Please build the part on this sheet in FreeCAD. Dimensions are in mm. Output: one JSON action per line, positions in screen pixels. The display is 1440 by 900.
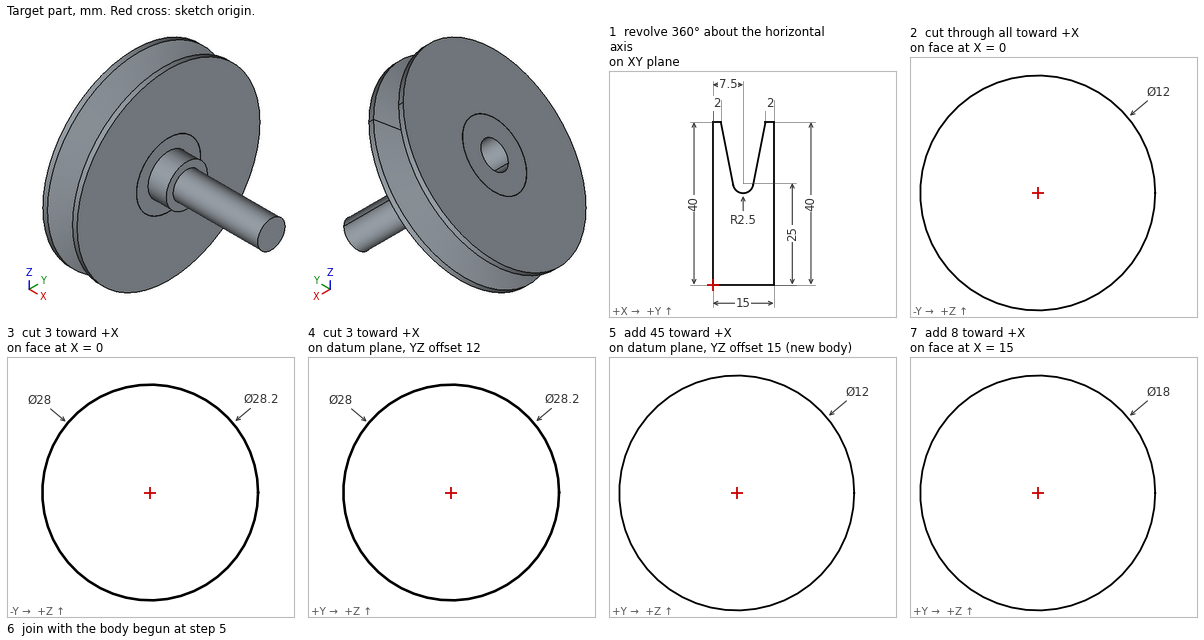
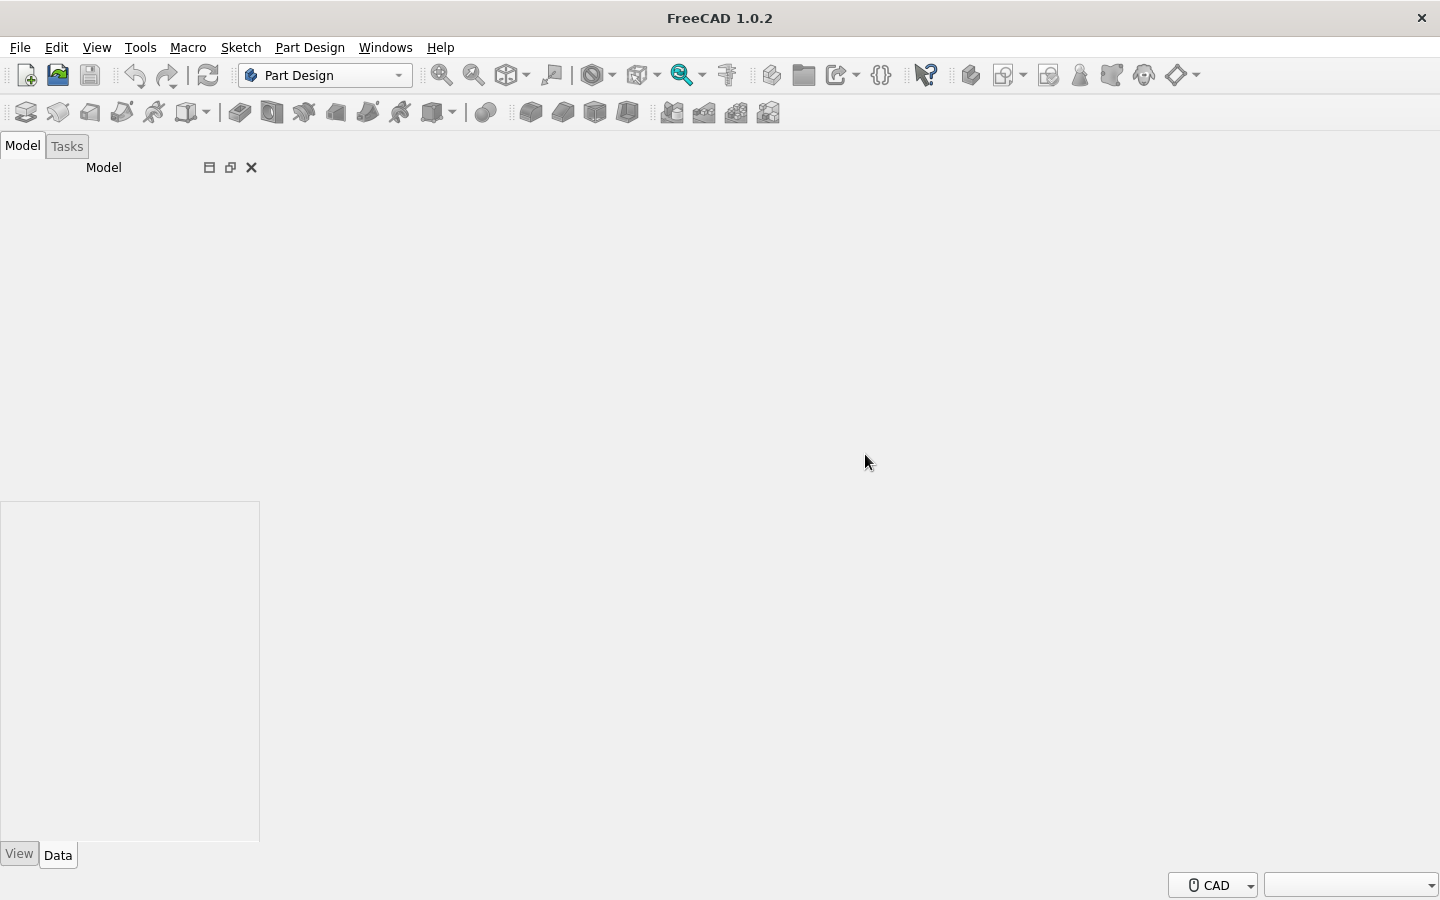
{"action": "left_click", "coordinate": [26, 76]}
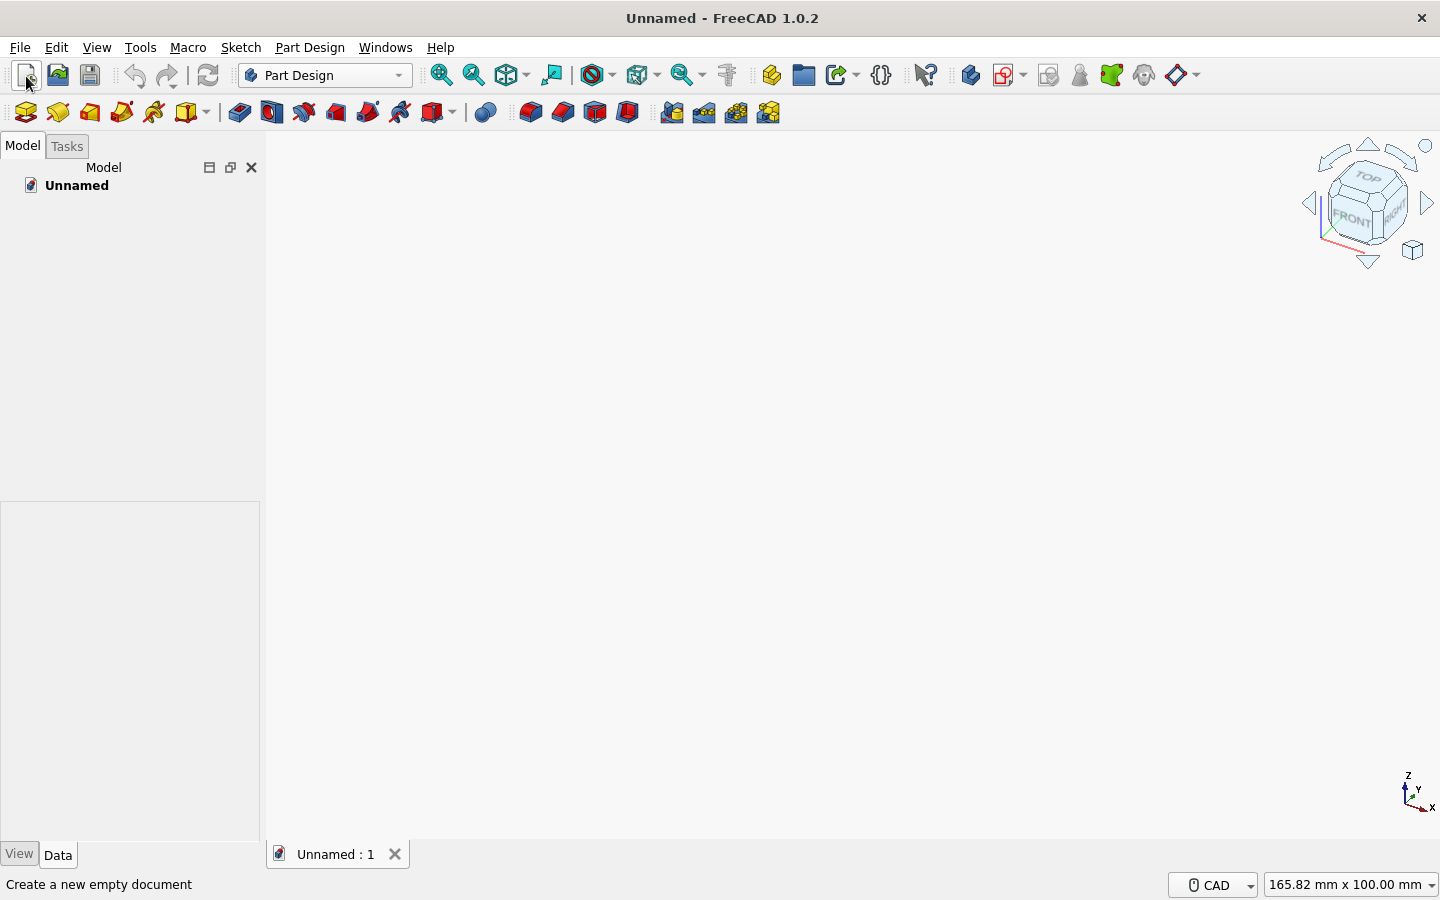
{"action": "left_click", "coordinate": [1004, 76]}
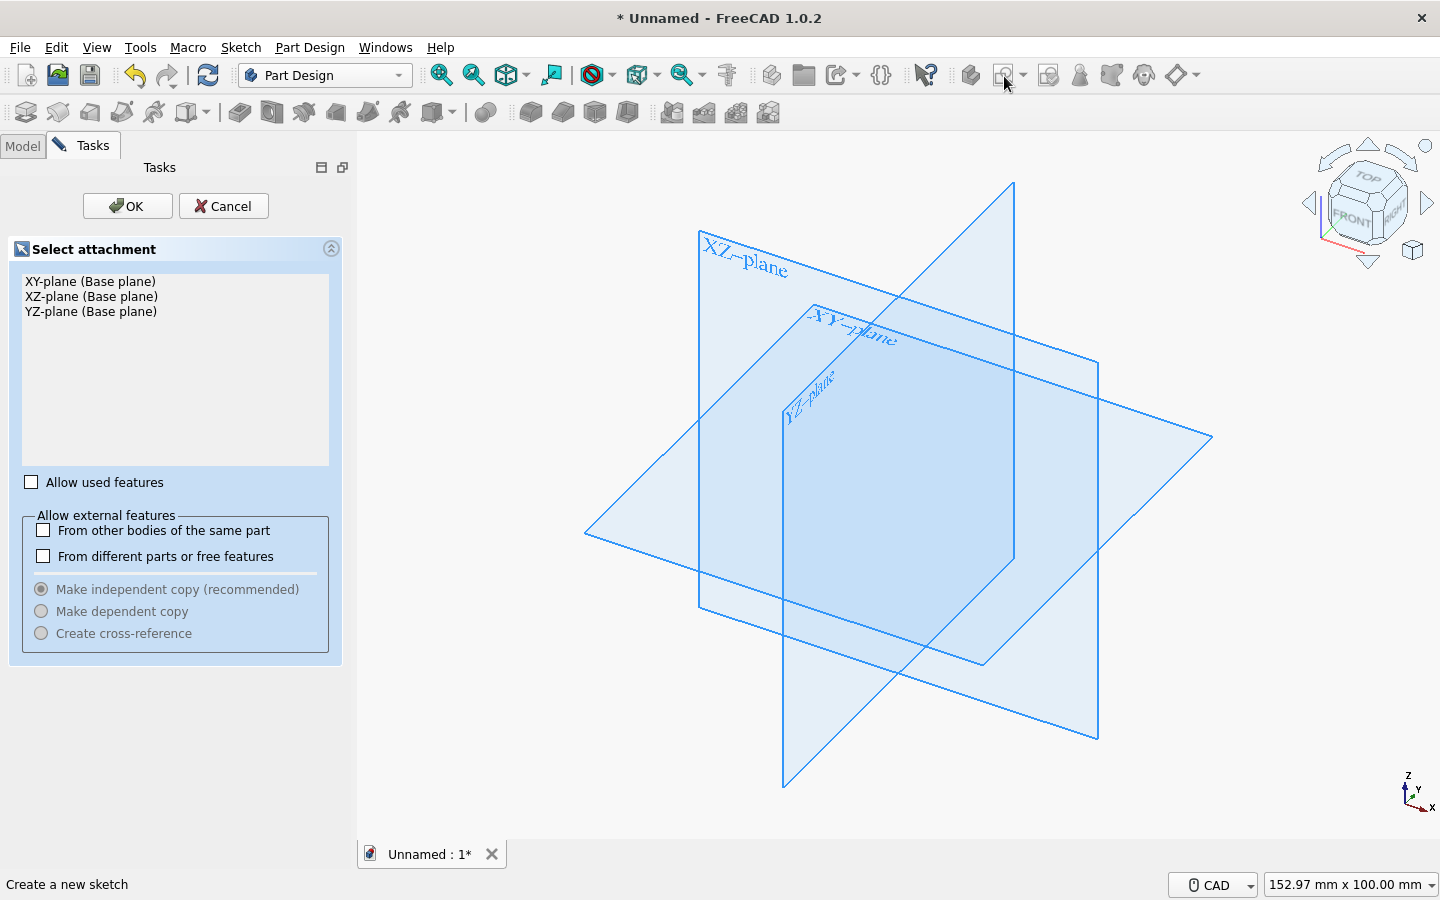
{"action": "left_click", "coordinate": [82, 282]}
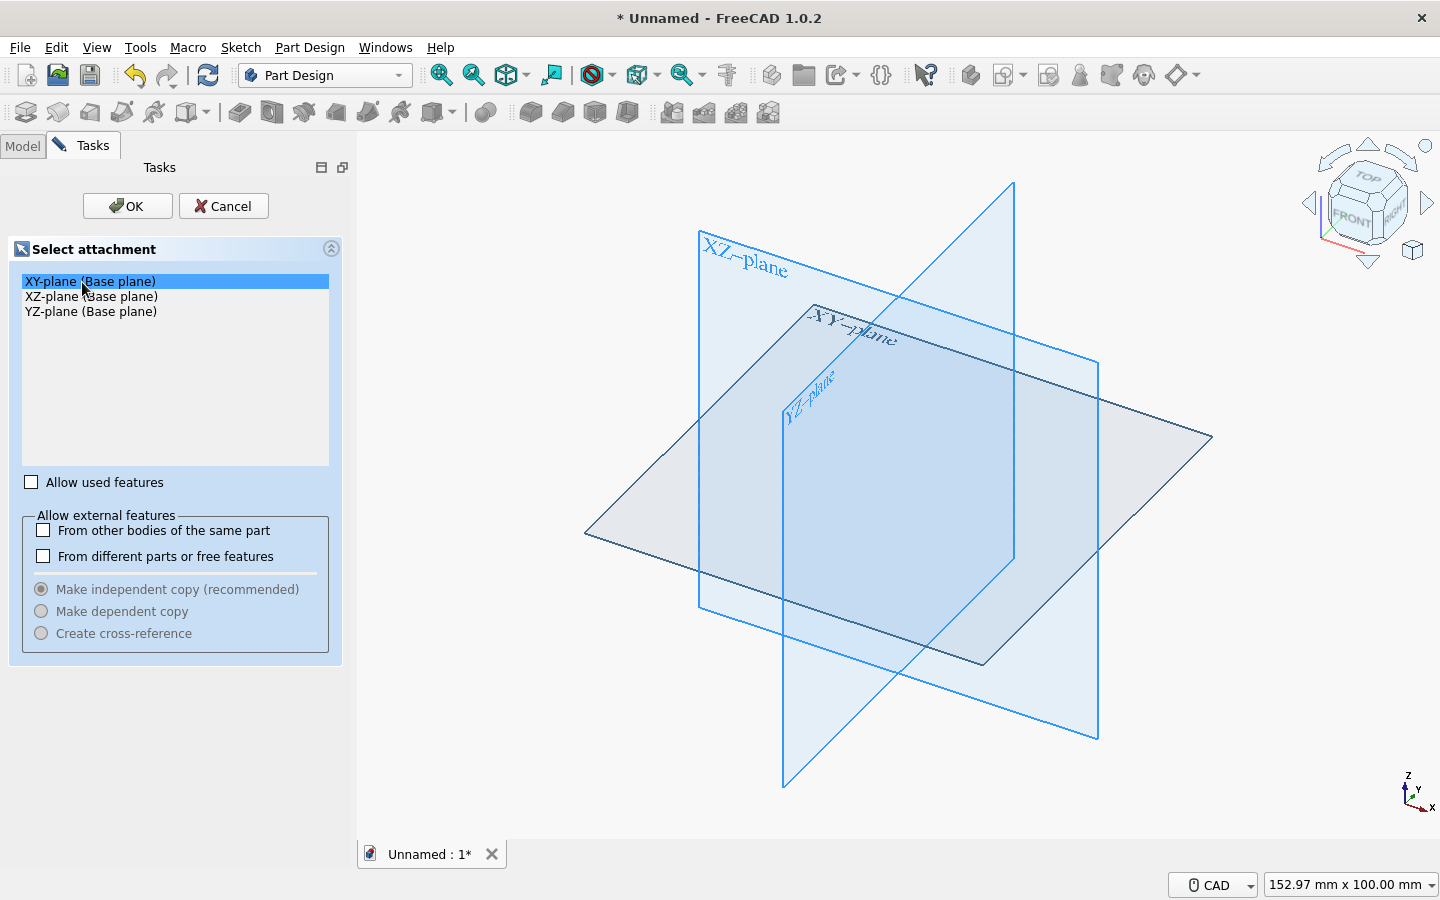
{"action": "left_click", "coordinate": [128, 206]}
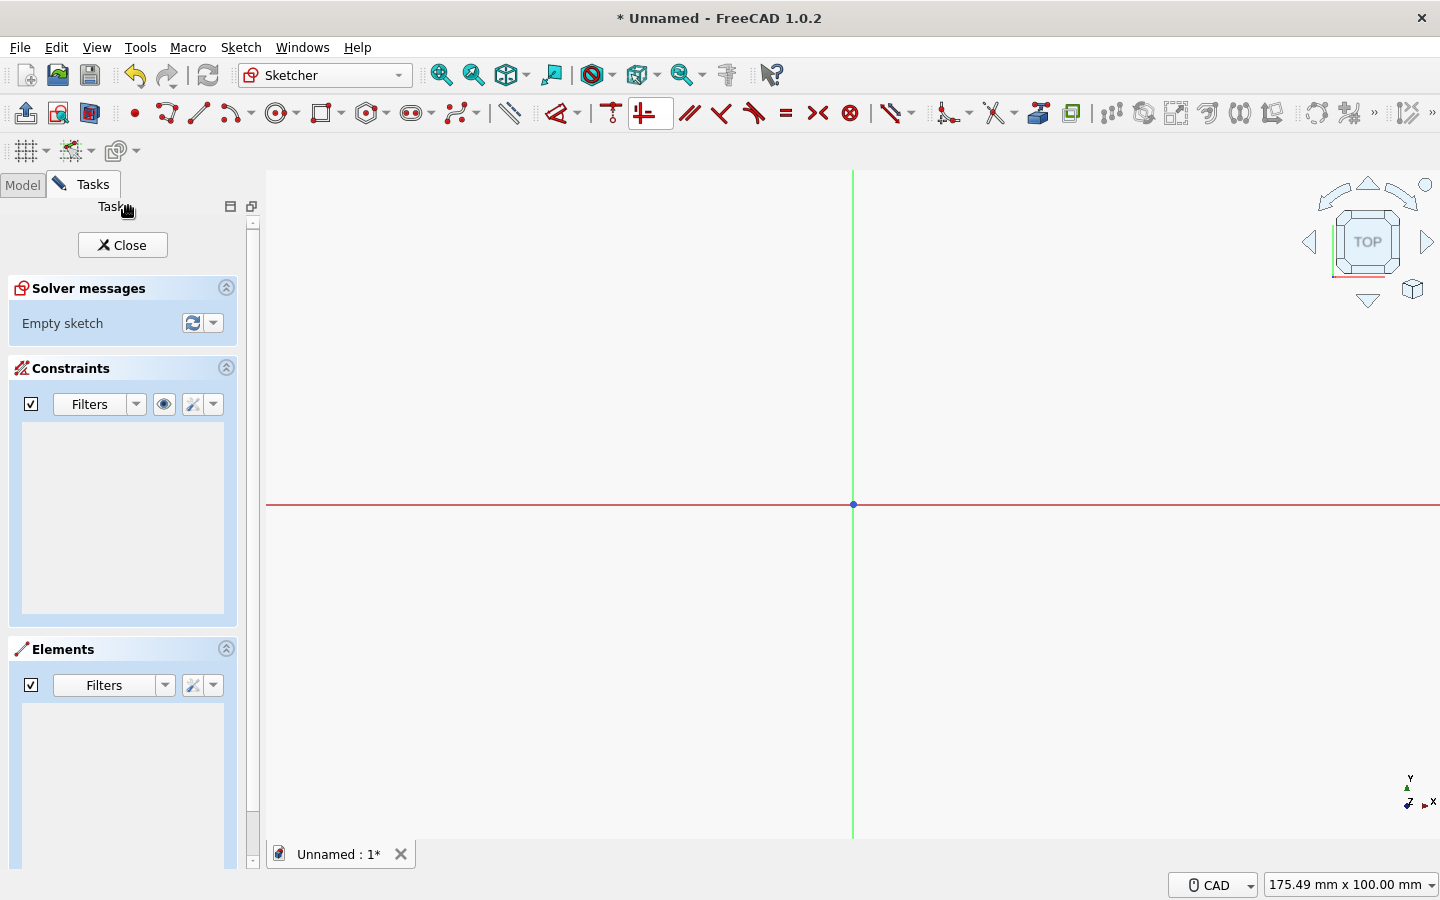
{"action": "scroll", "coordinate": [1144, 198], "scroll_direction": "up", "scroll_amount": 2}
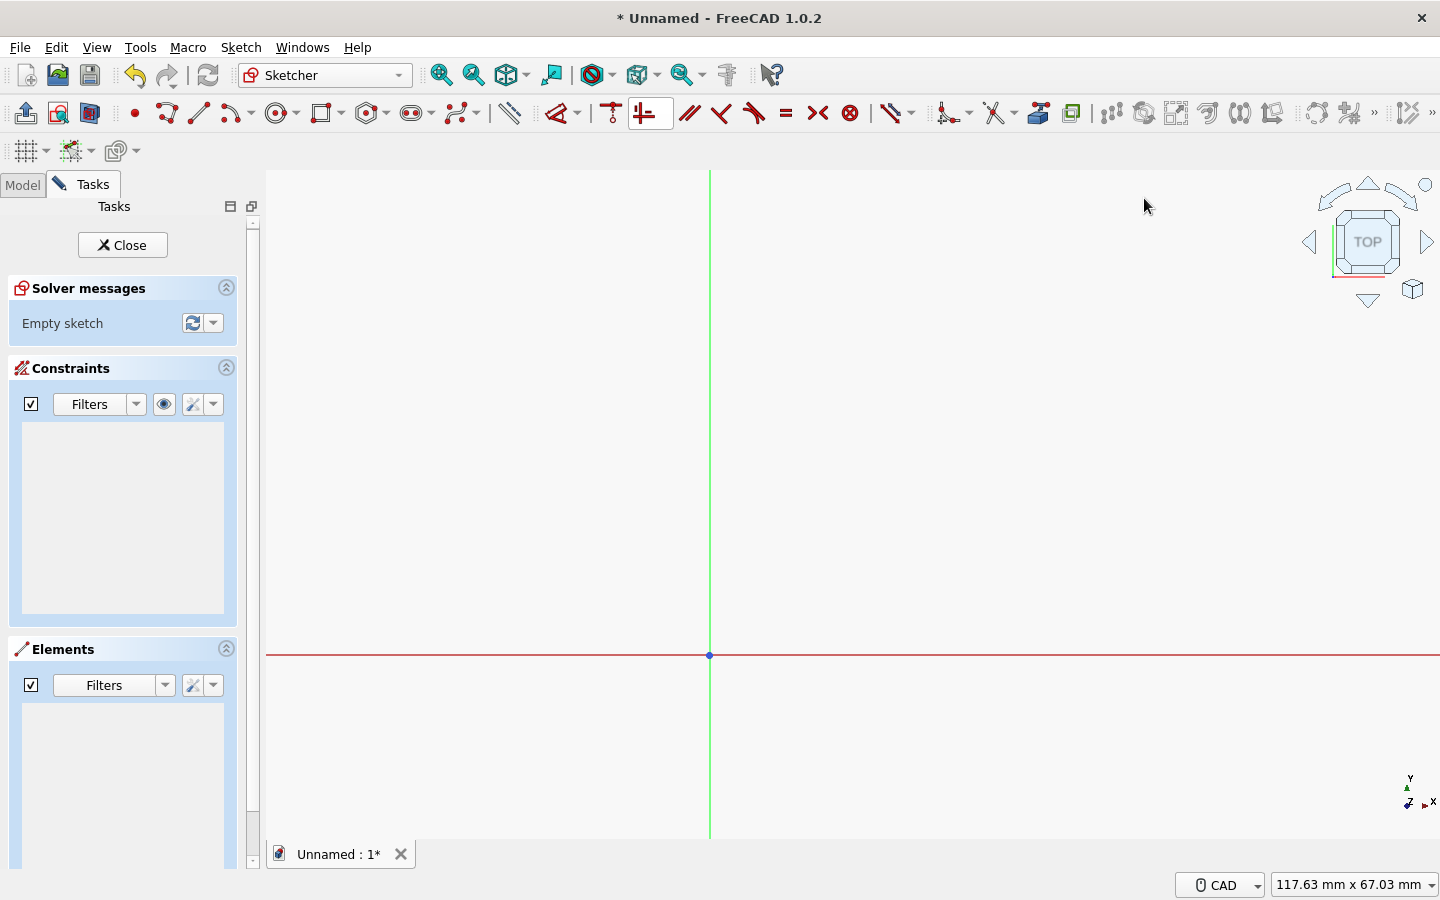
{"action": "left_click", "coordinate": [168, 114]}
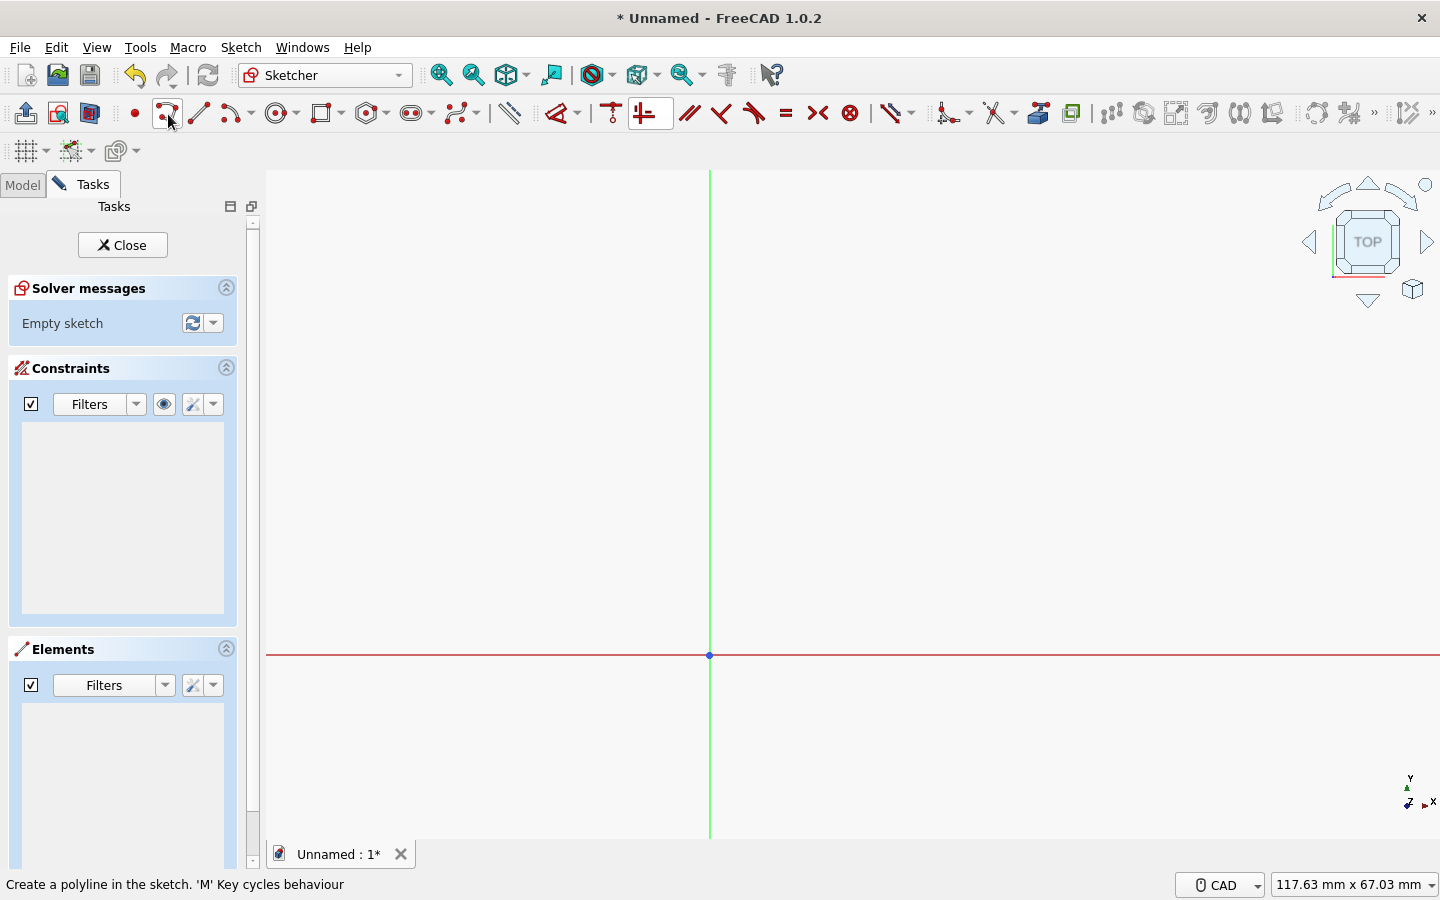
{"action": "left_click", "coordinate": [760, 411]}
{"action": "left_click", "coordinate": [729, 256]}
{"action": "left_click", "coordinate": [710, 256]}
{"action": "left_click", "coordinate": [710, 655]}
{"action": "left_click", "coordinate": [859, 646]}
{"action": "left_click", "coordinate": [859, 256]}
{"action": "left_click", "coordinate": [839, 256]}
{"action": "left_click", "coordinate": [809, 411]}
{"action": "right_click", "coordinate": [809, 411]}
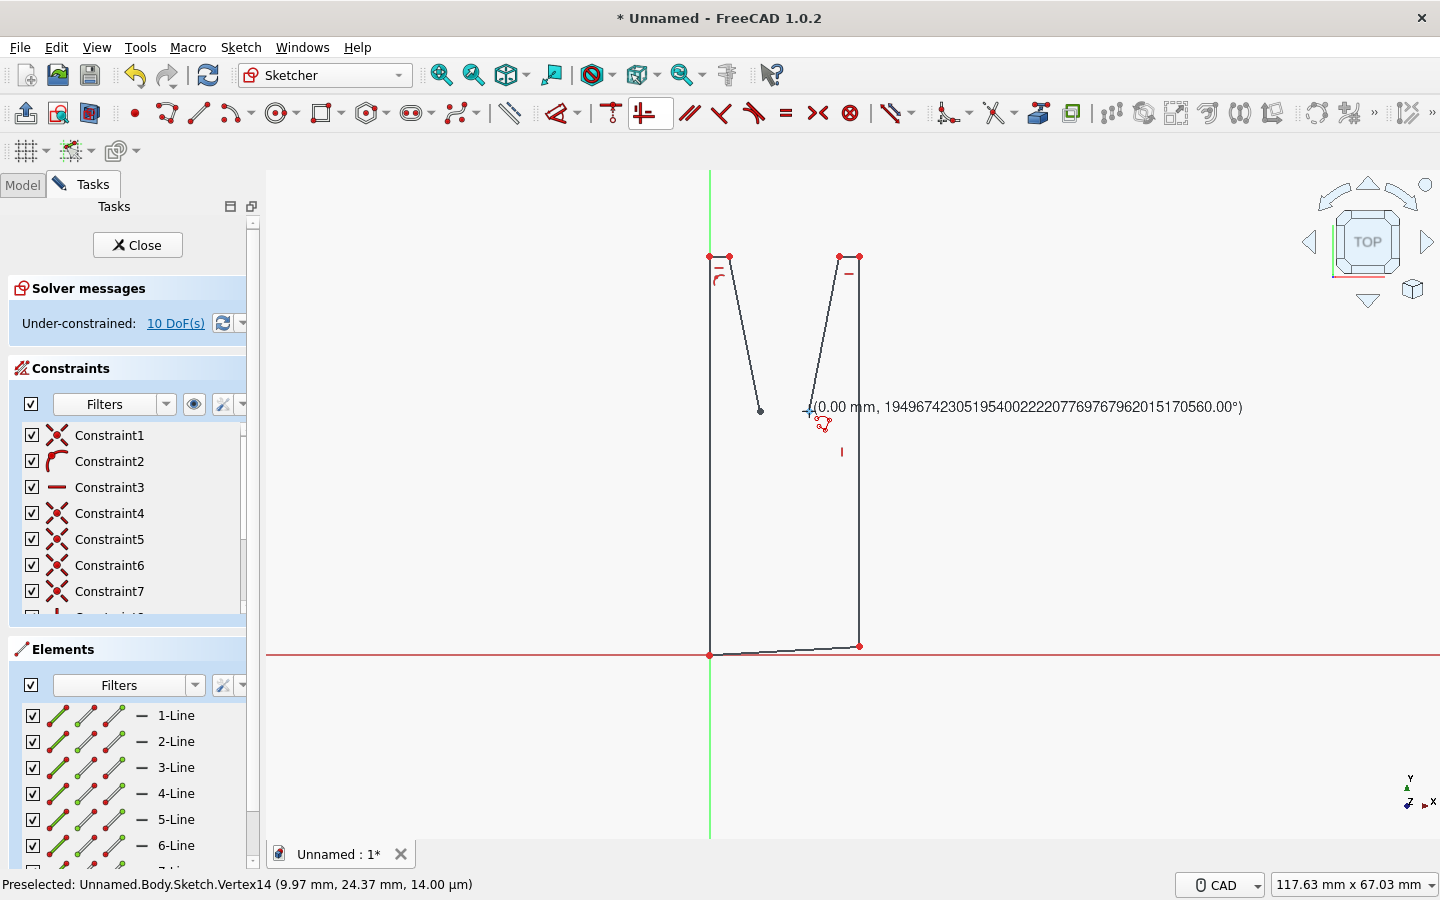
{"action": "key", "text": "g 3 a"}